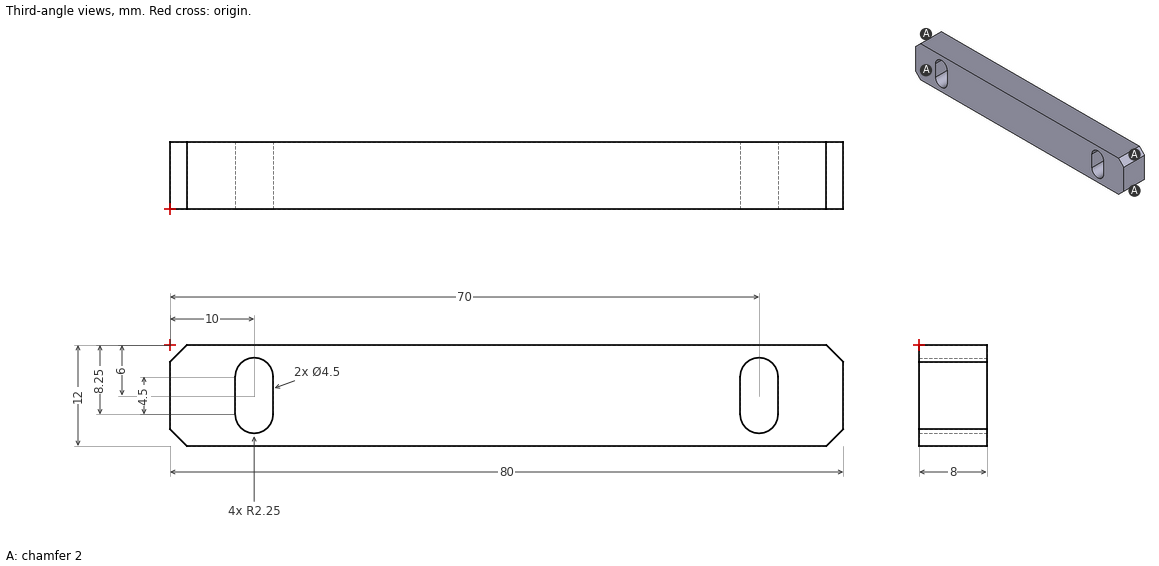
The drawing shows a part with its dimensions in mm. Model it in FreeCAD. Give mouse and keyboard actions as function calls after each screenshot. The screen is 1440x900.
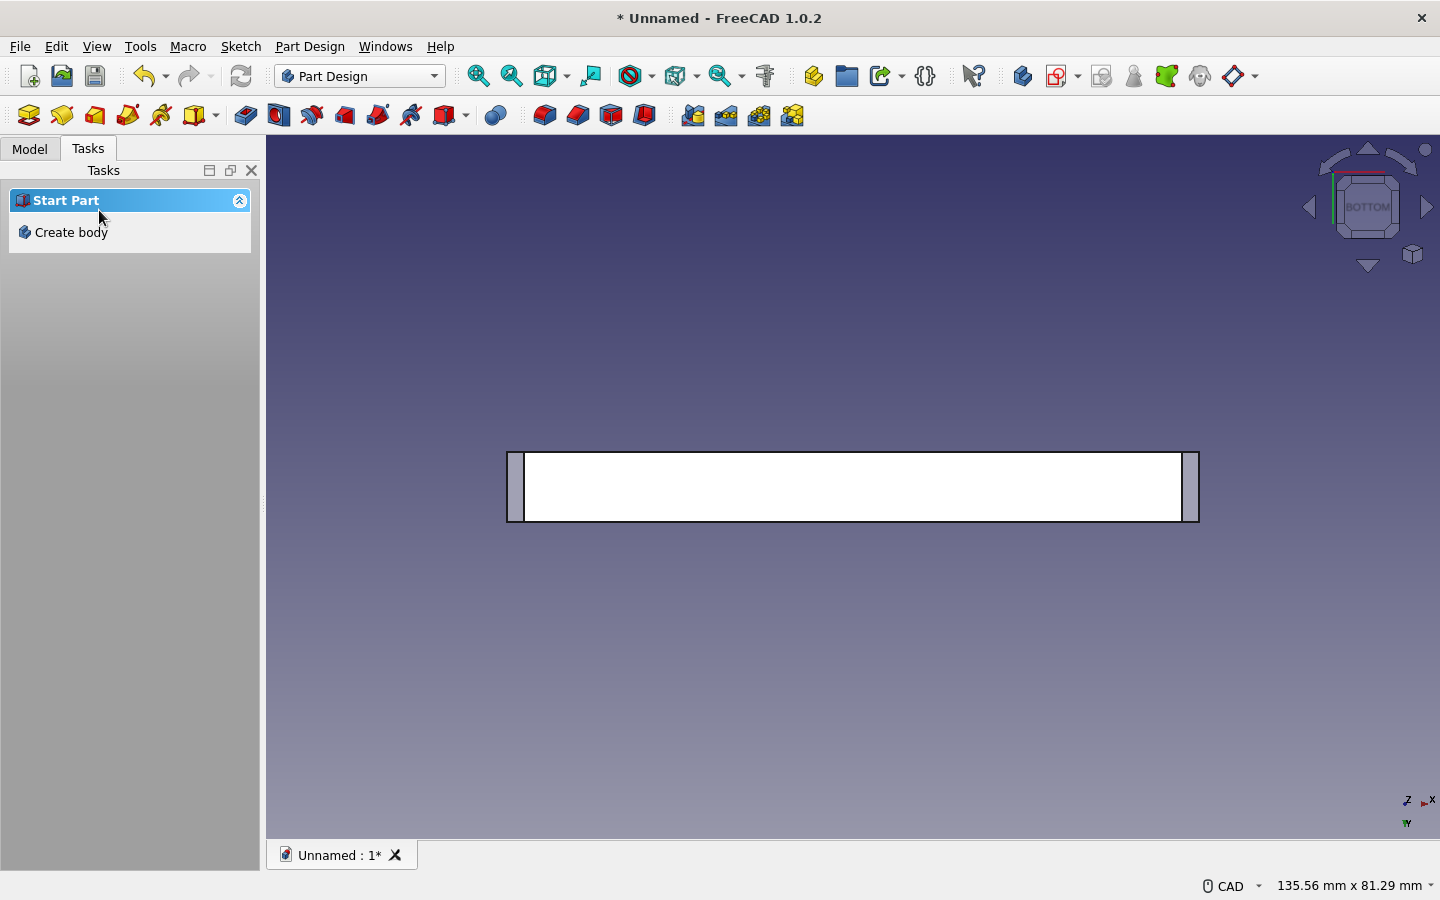
key(0)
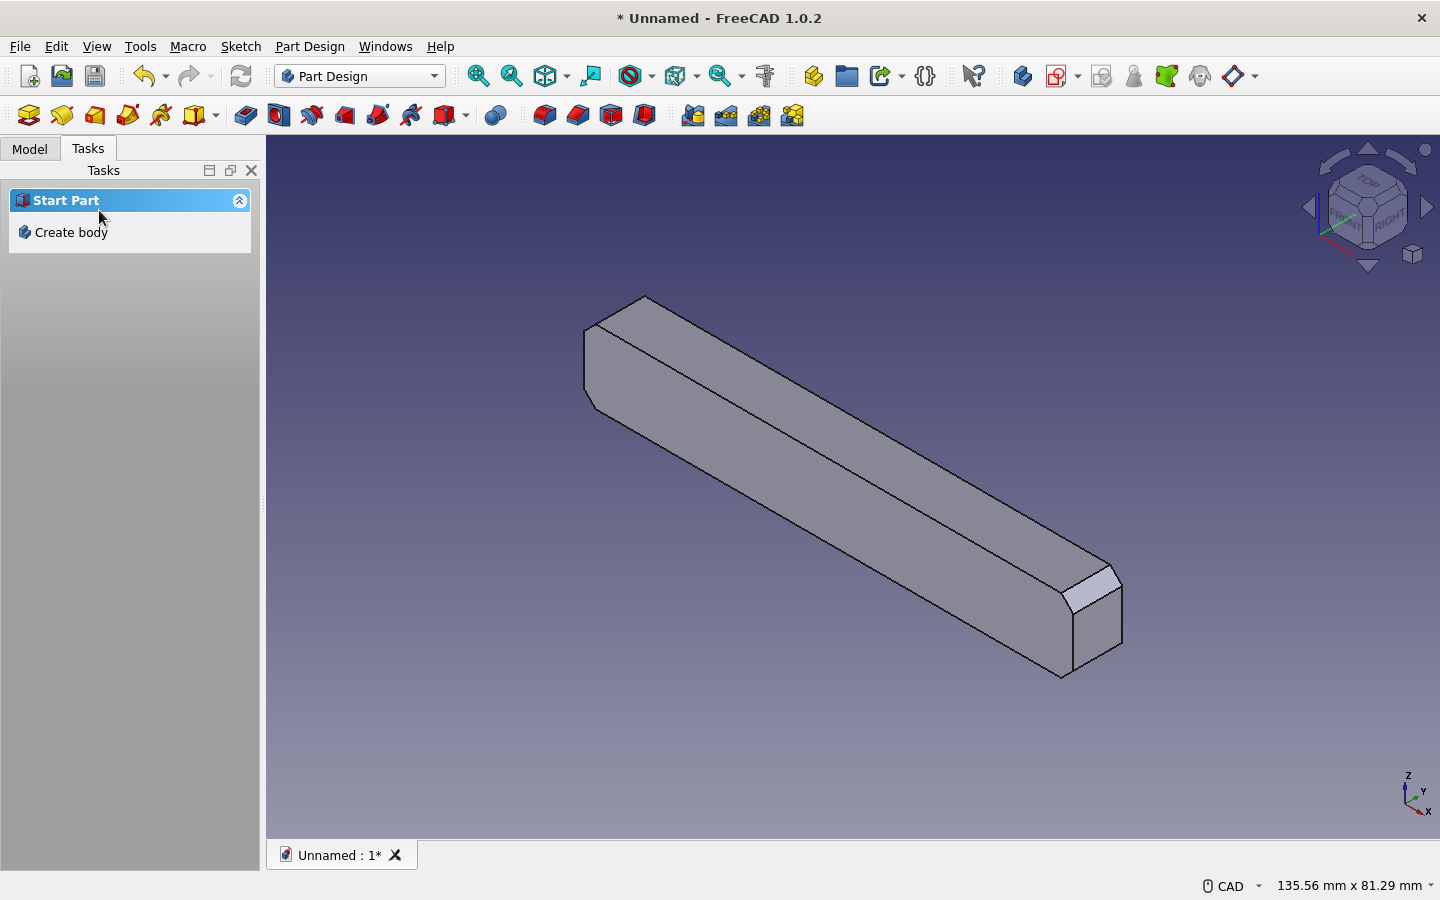
click(968, 581)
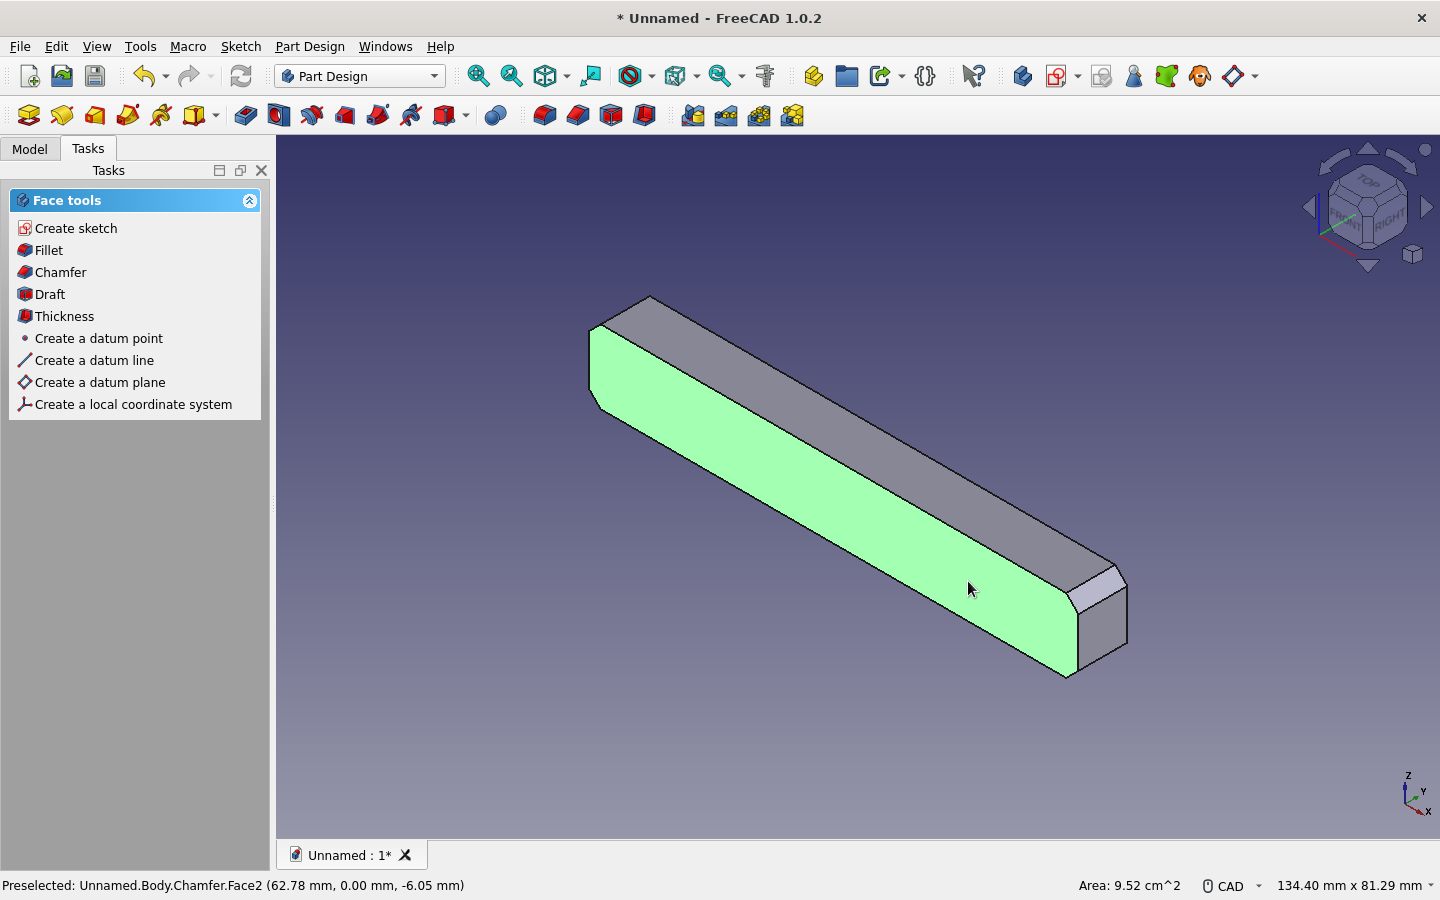
click(1056, 76)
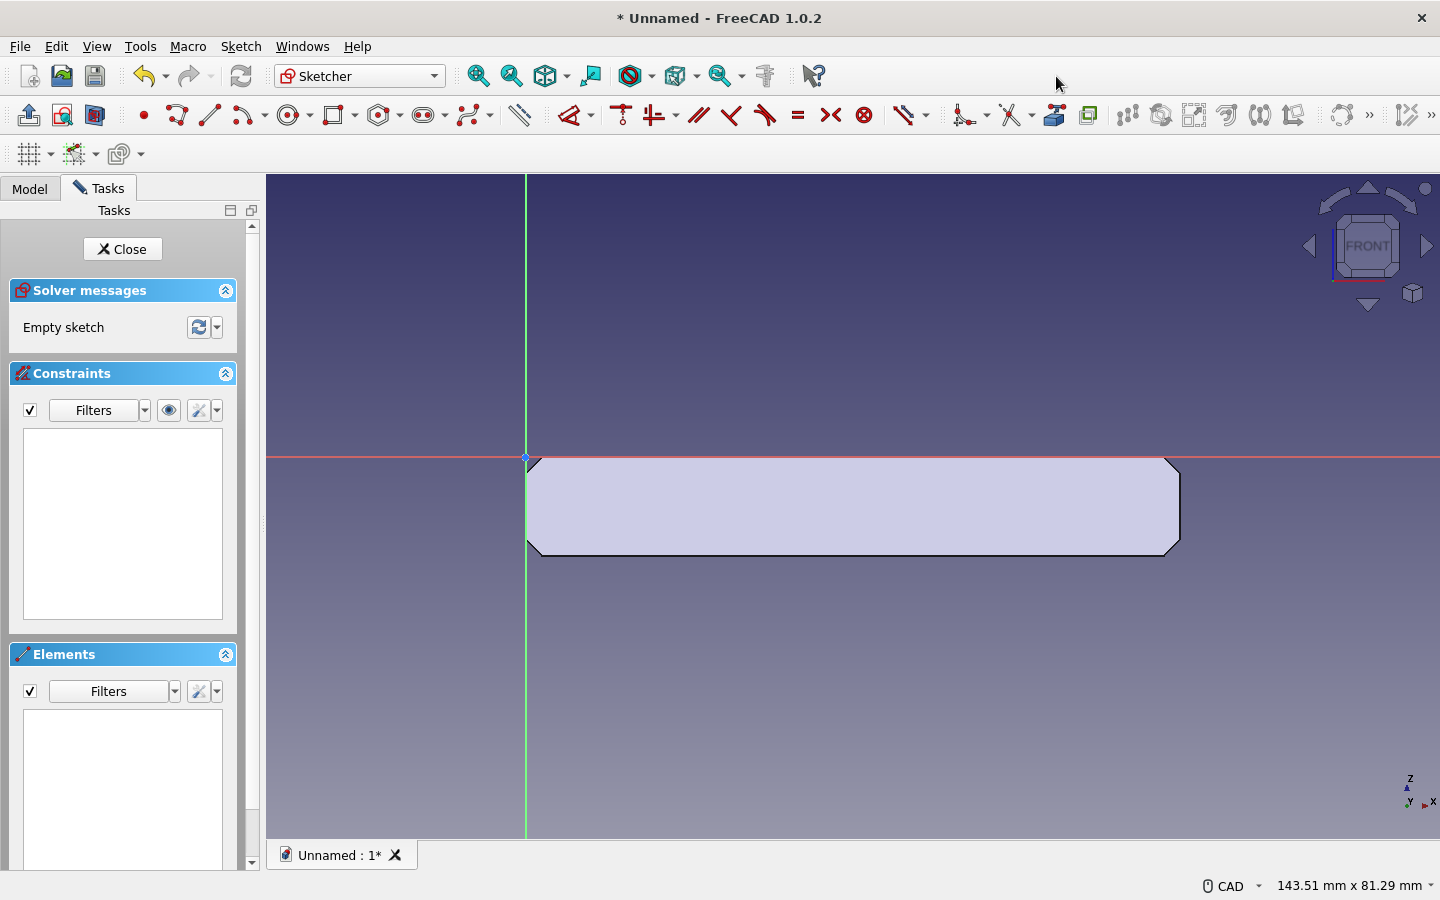
key(g)
key(c)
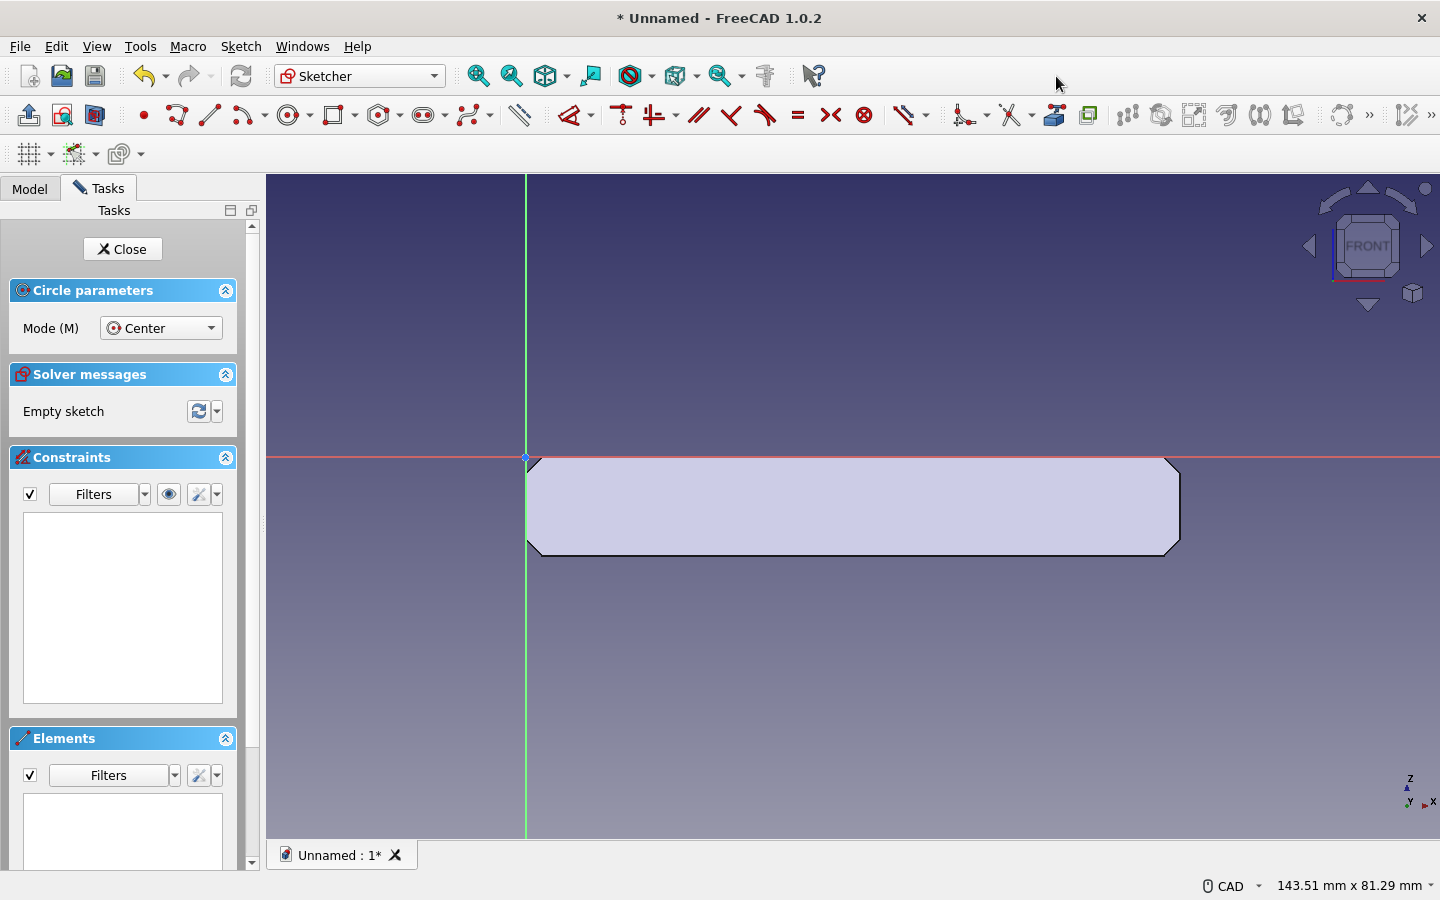
scroll(608, 506, up, 2)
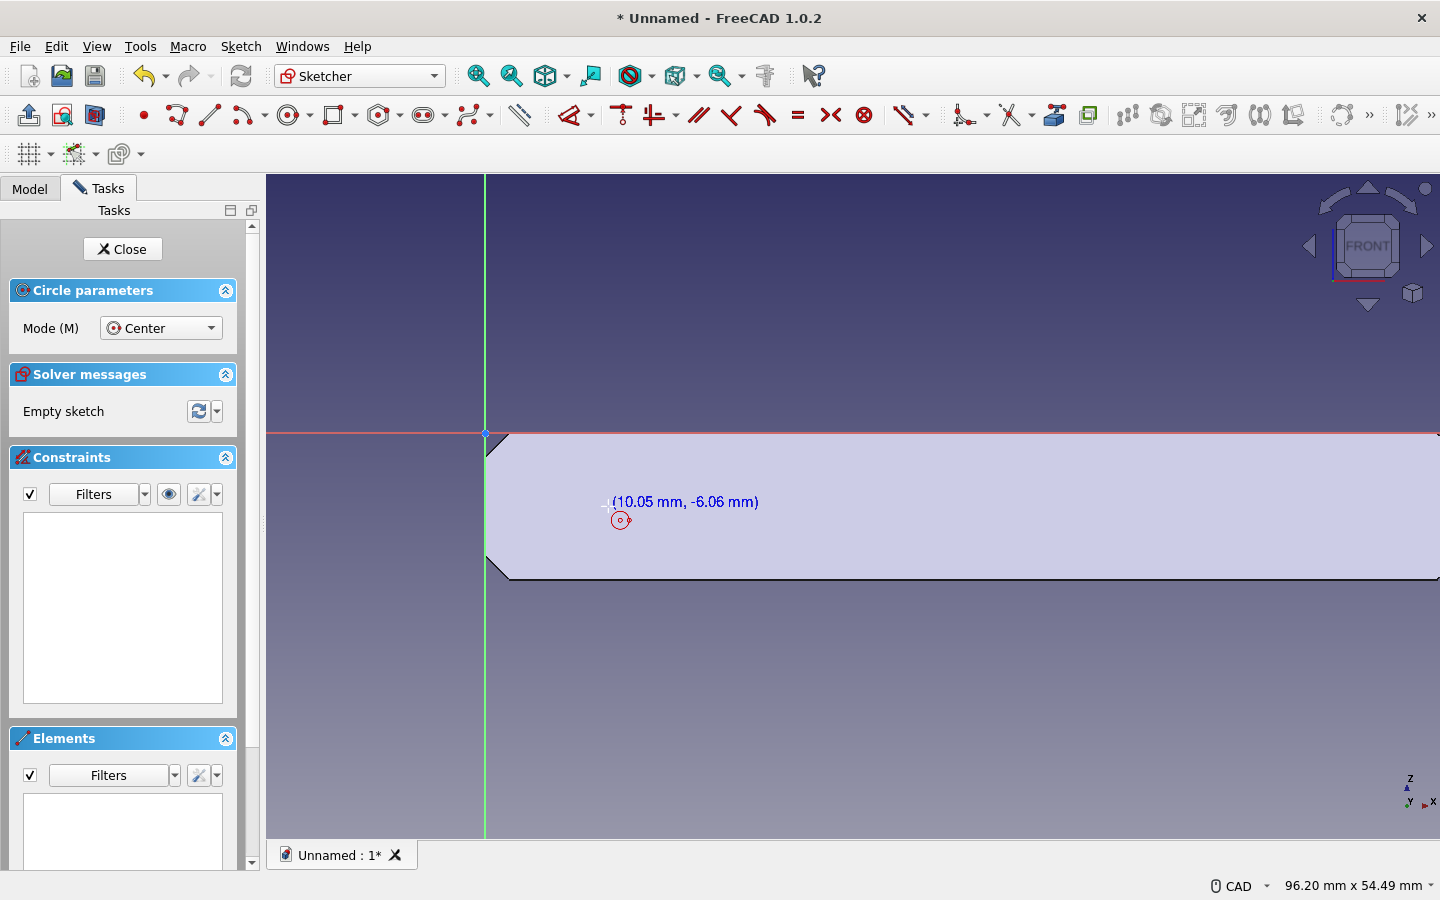
click(607, 506)
click(627, 487)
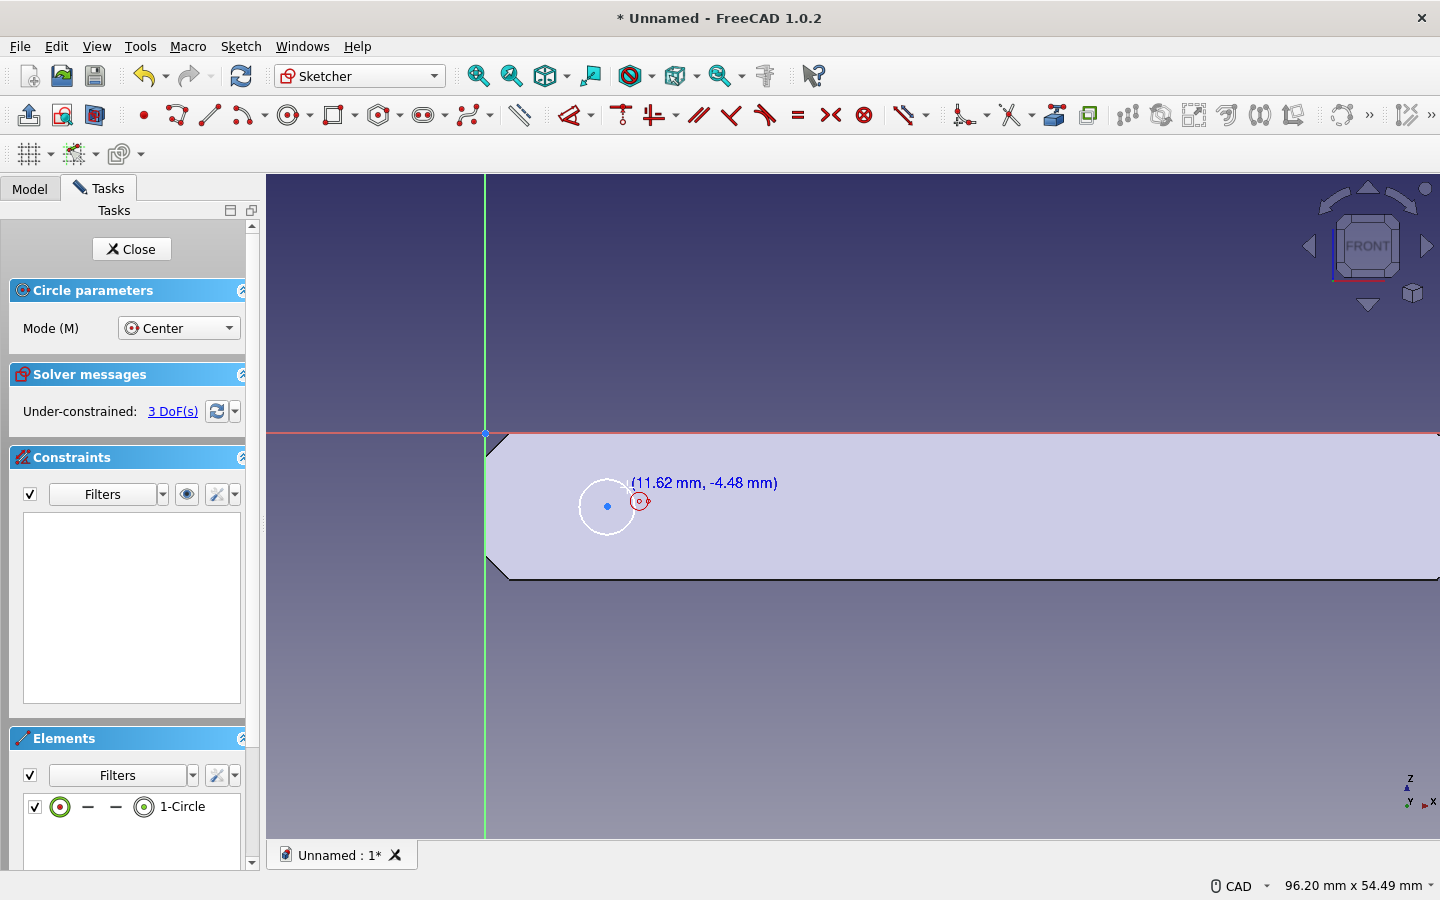
scroll(294, 610, down, 1)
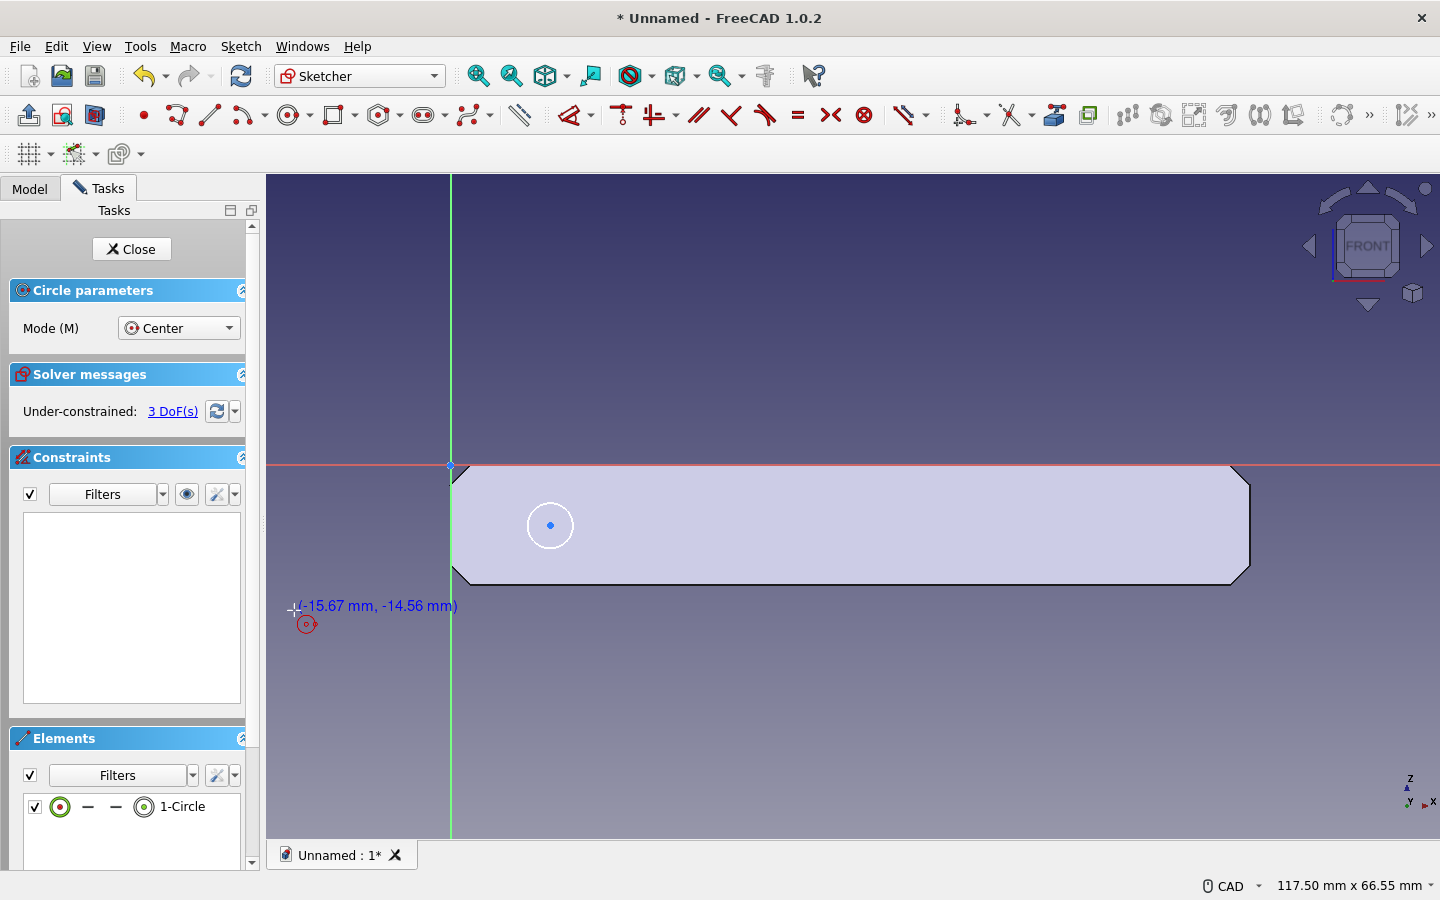
click(1150, 525)
click(1166, 509)
key(Escape)